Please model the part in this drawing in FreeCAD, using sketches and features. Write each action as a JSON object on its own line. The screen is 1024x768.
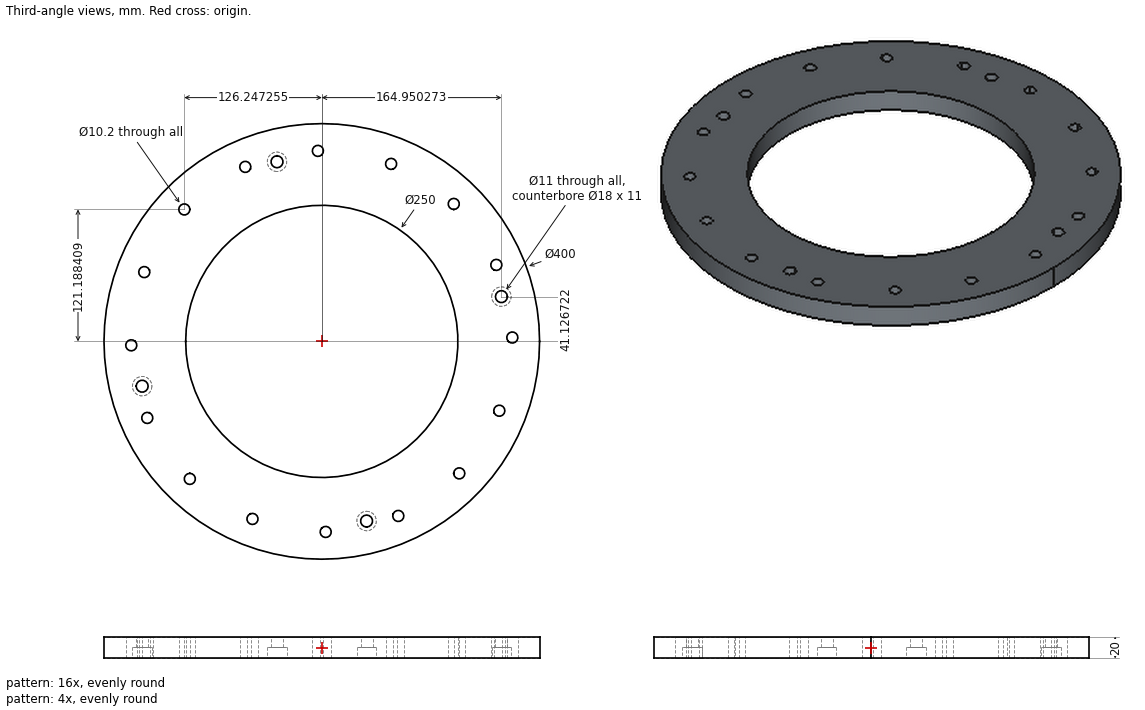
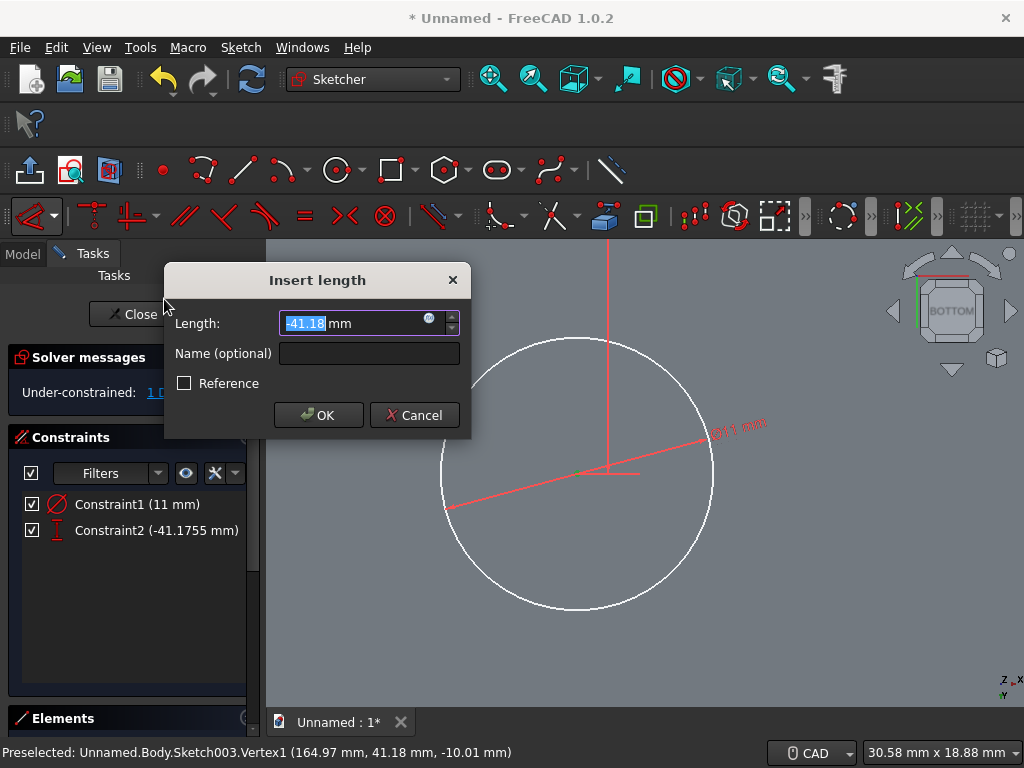
{"action": "type", "text": "-41.126722"}
{"action": "key", "text": "Return"}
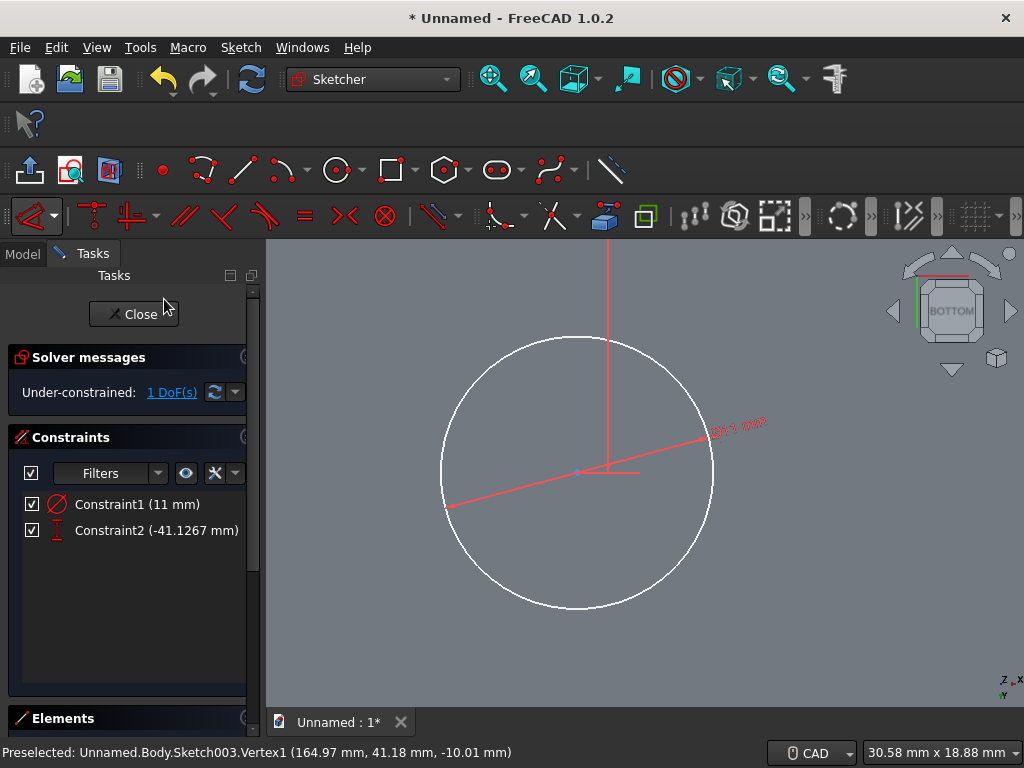
{"action": "left_click", "coordinate": [577, 473]}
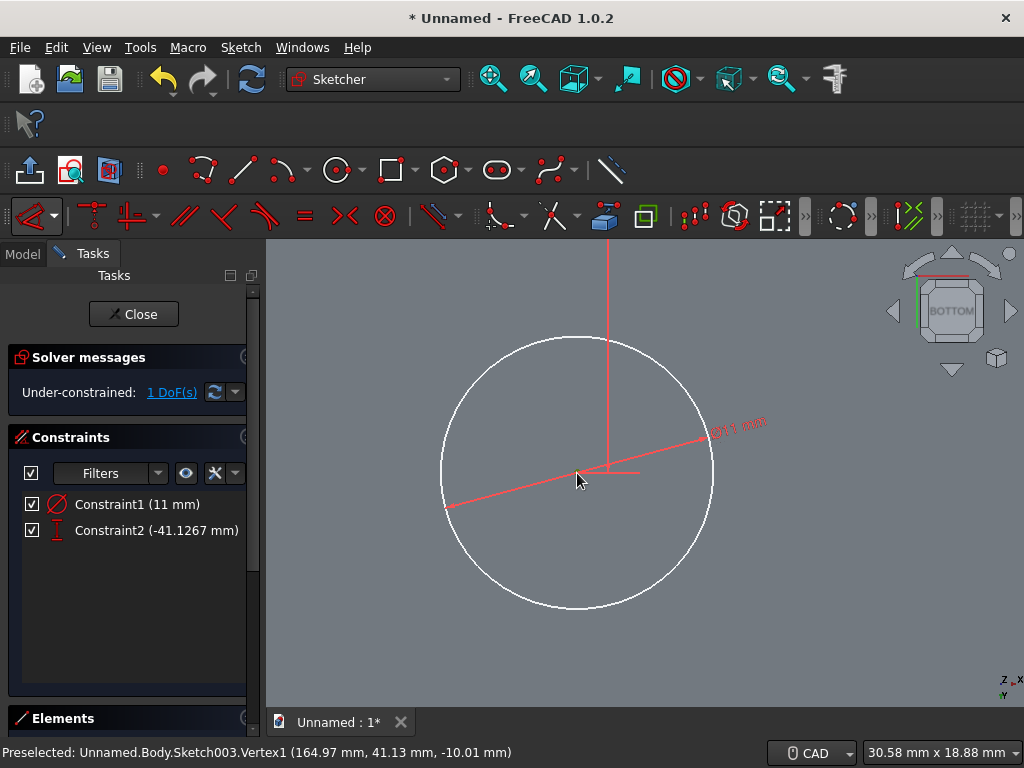
{"action": "key", "text": "l"}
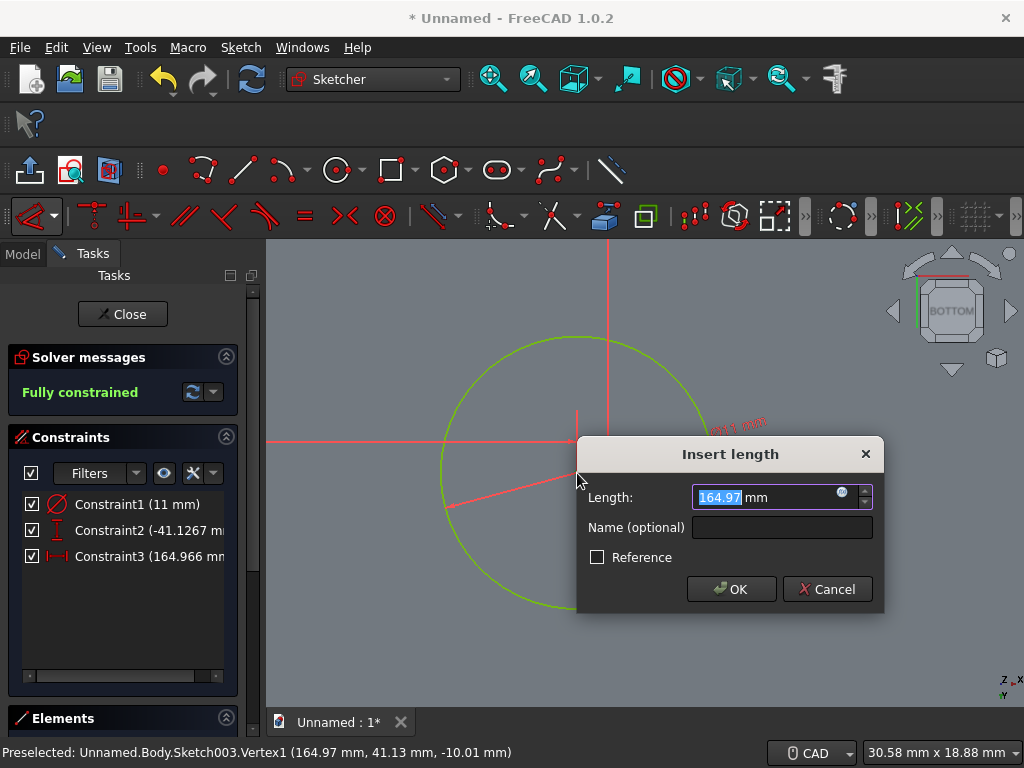
{"action": "type", "text": "164.950273"}
{"action": "key", "text": "Return"}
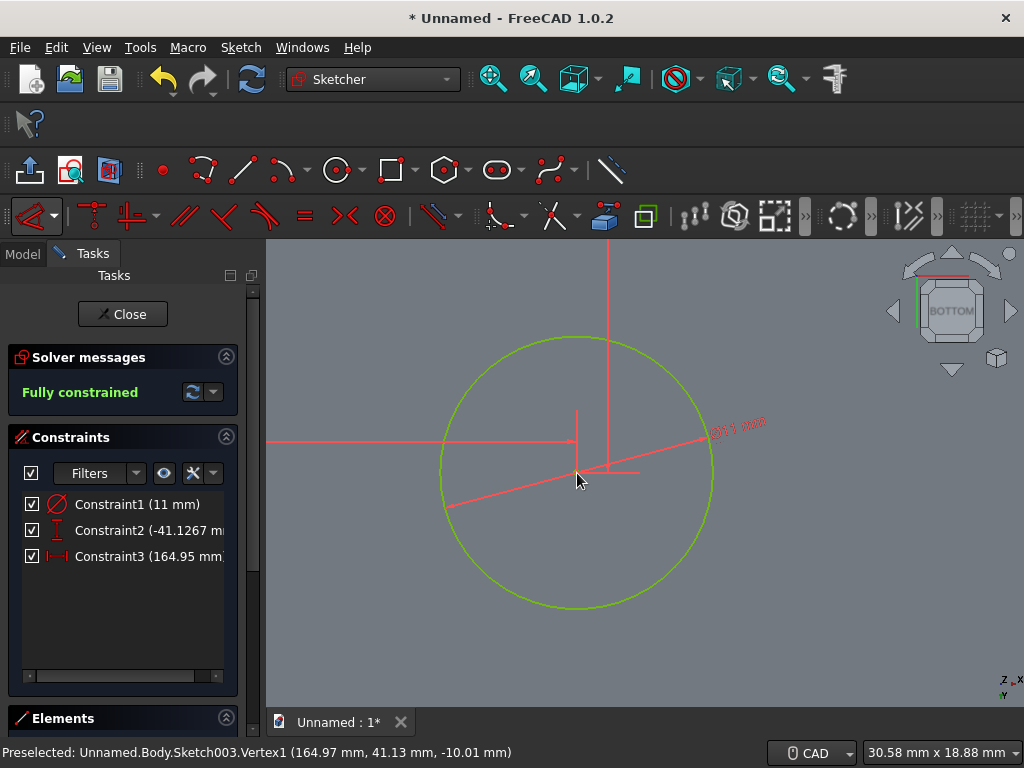
{"action": "left_click", "coordinate": [123, 314]}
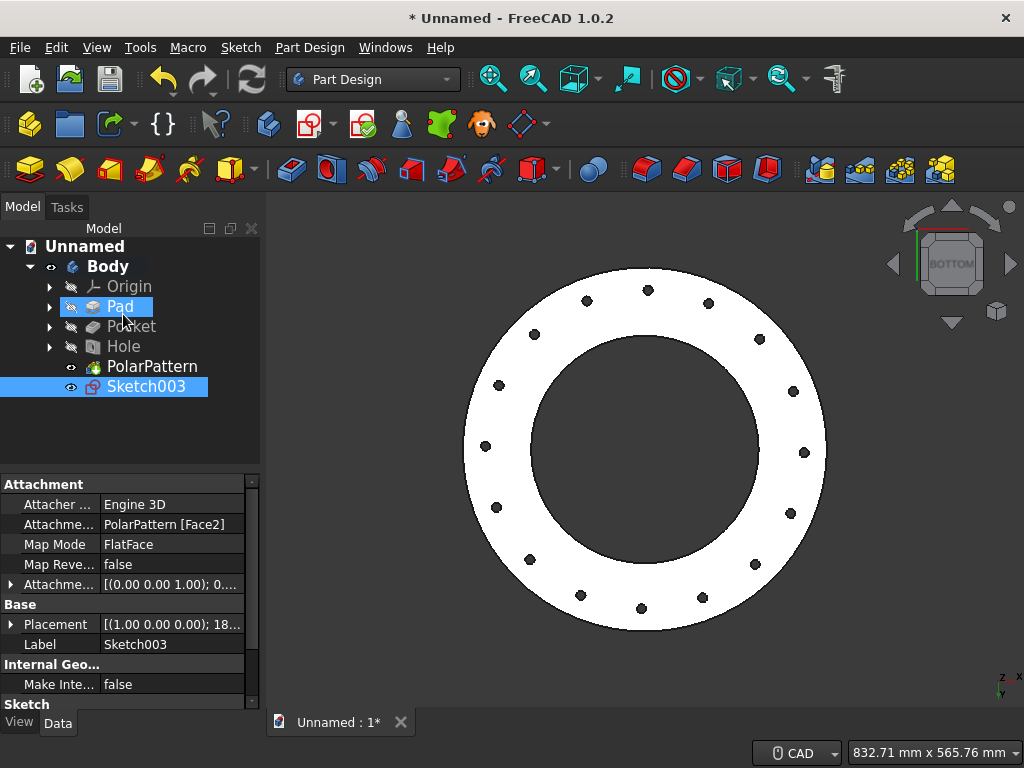
{"action": "left_click", "coordinate": [332, 170]}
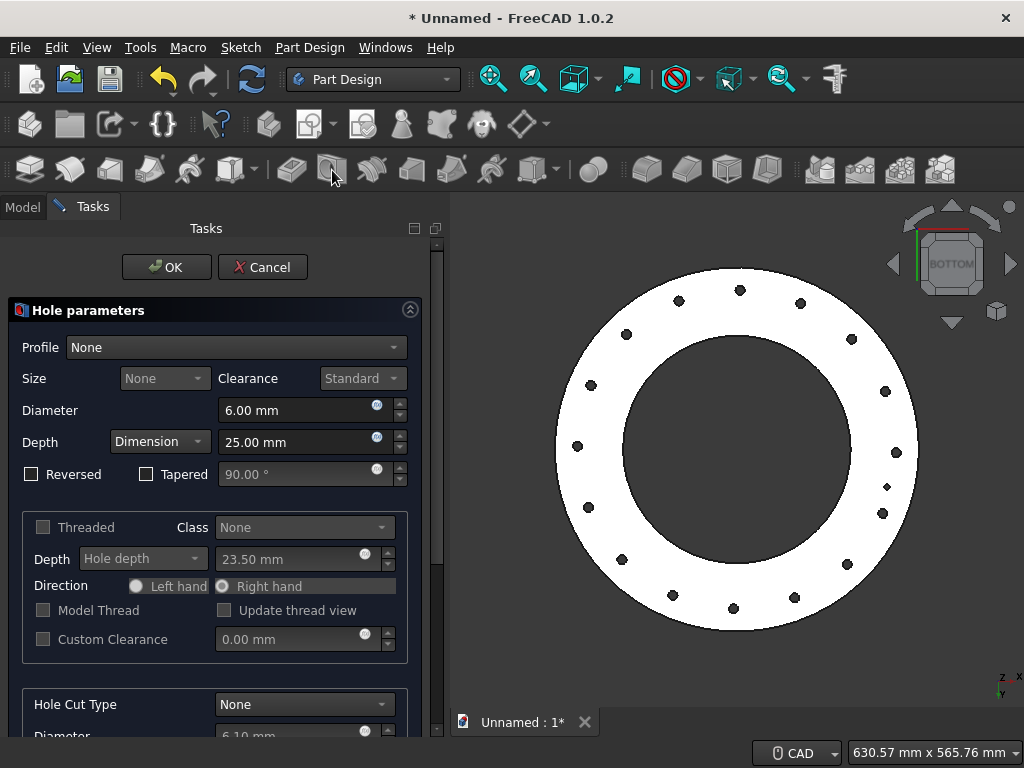
{"action": "triple_click", "coordinate": [305, 410]}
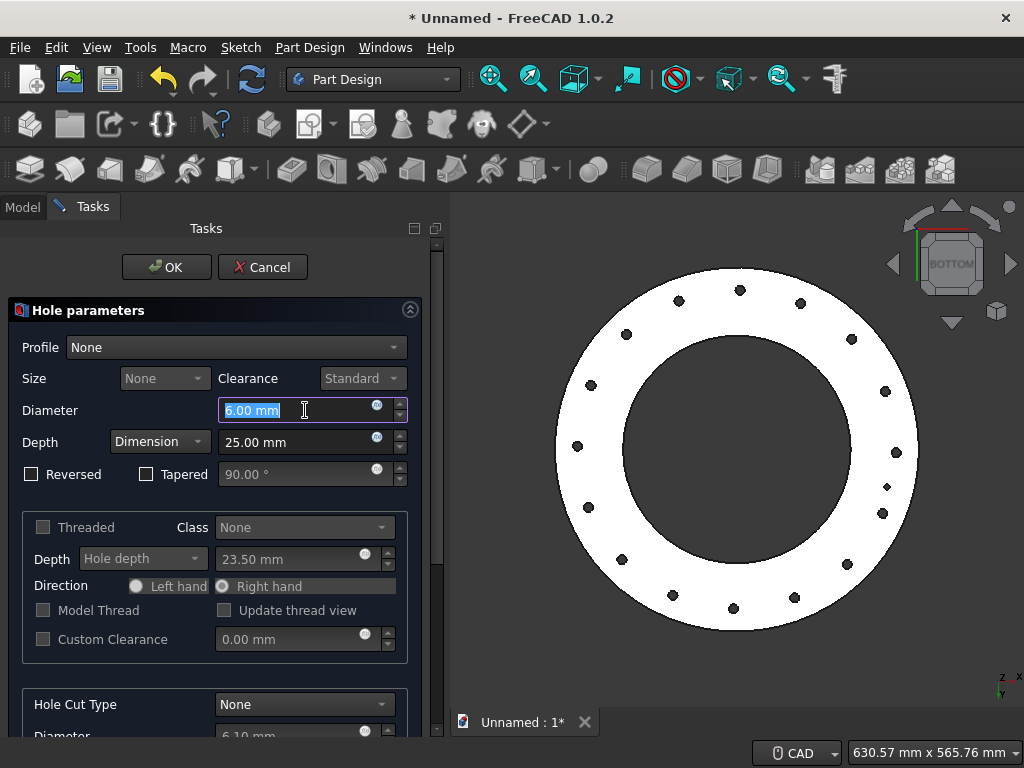
{"action": "type", "text": "11"}
{"action": "key", "text": "Tab"}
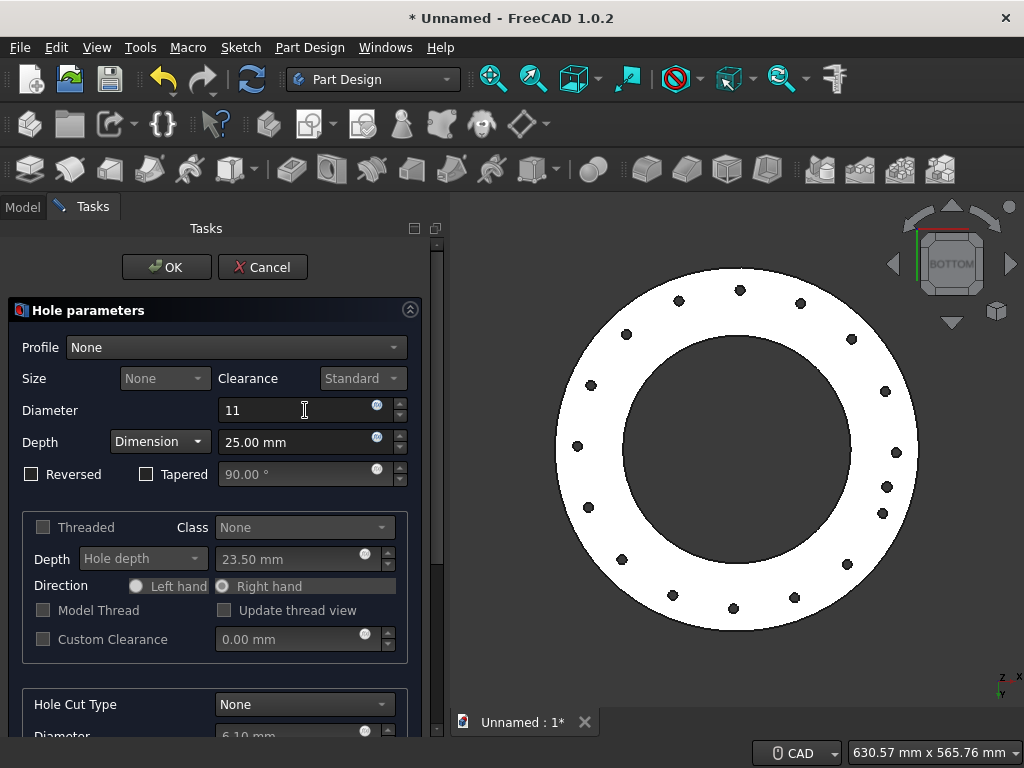
{"action": "left_click", "coordinate": [161, 442]}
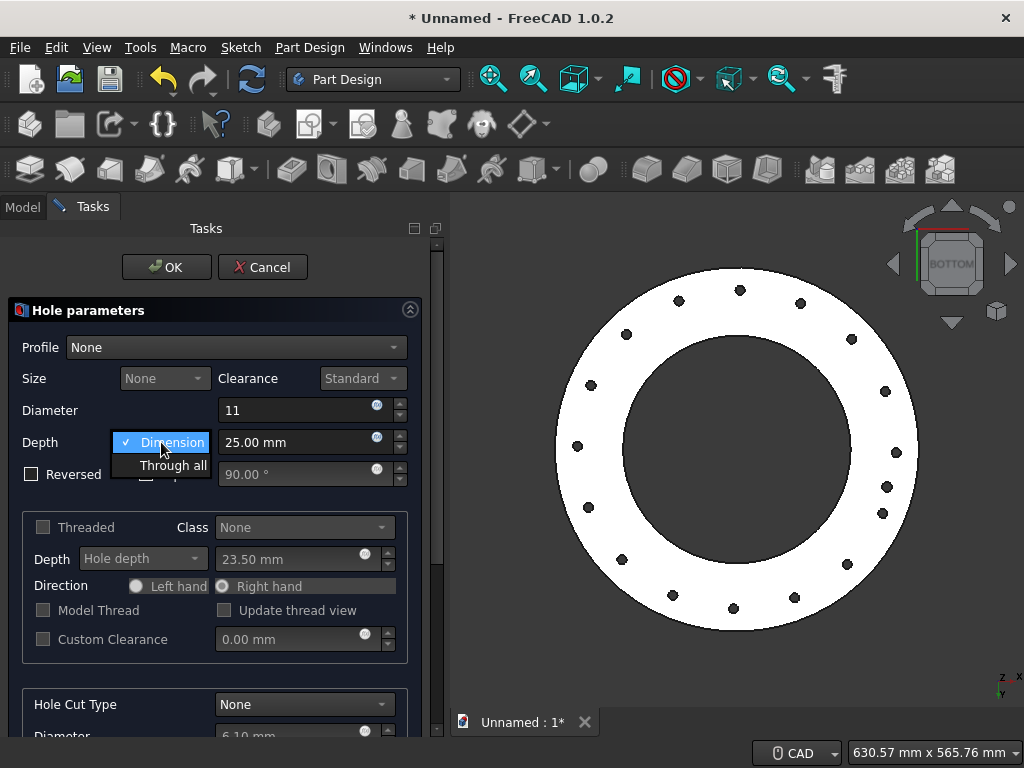
{"action": "left_click", "coordinate": [160, 466]}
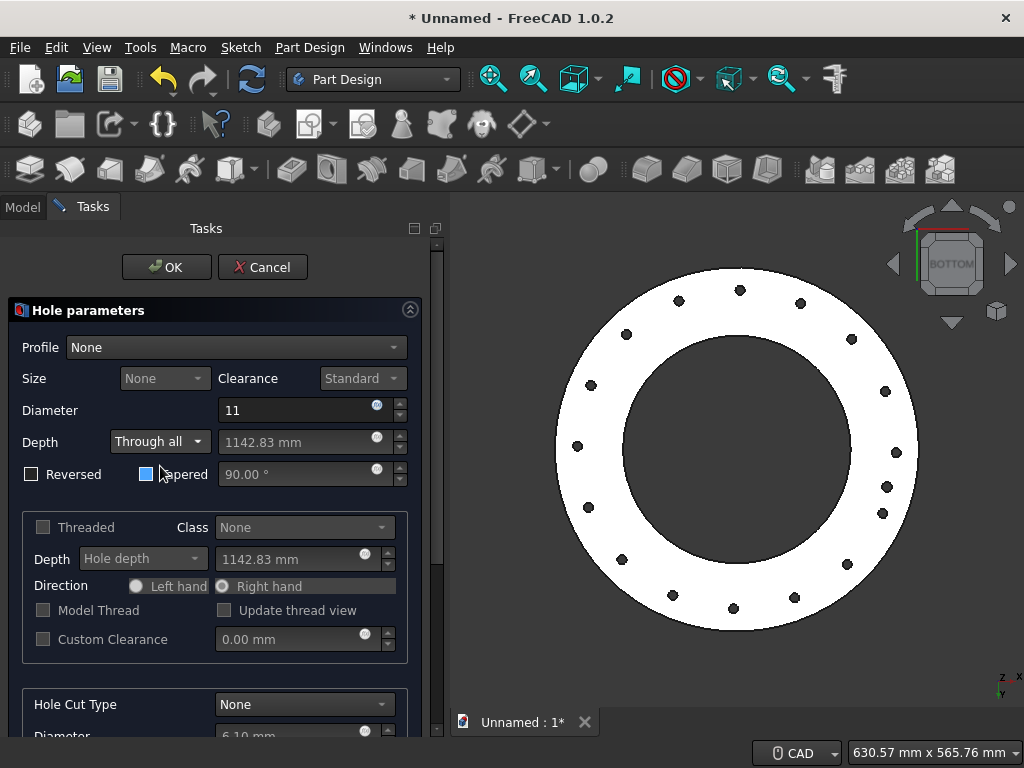
{"action": "left_click", "coordinate": [306, 704]}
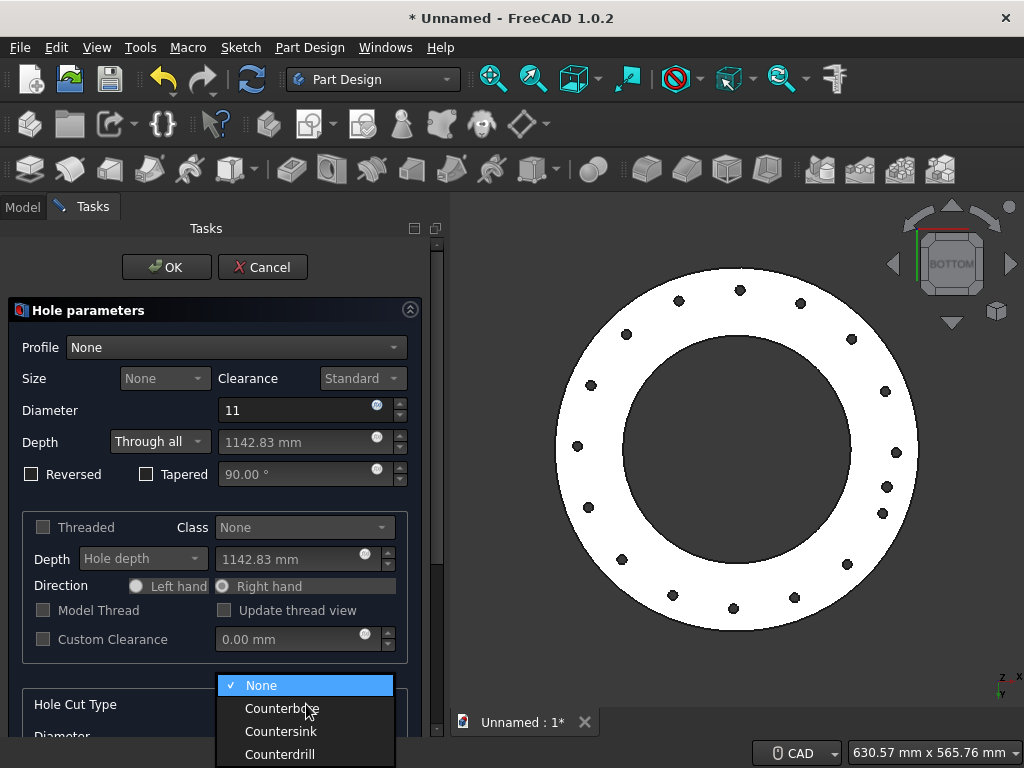
{"action": "left_click", "coordinate": [304, 708]}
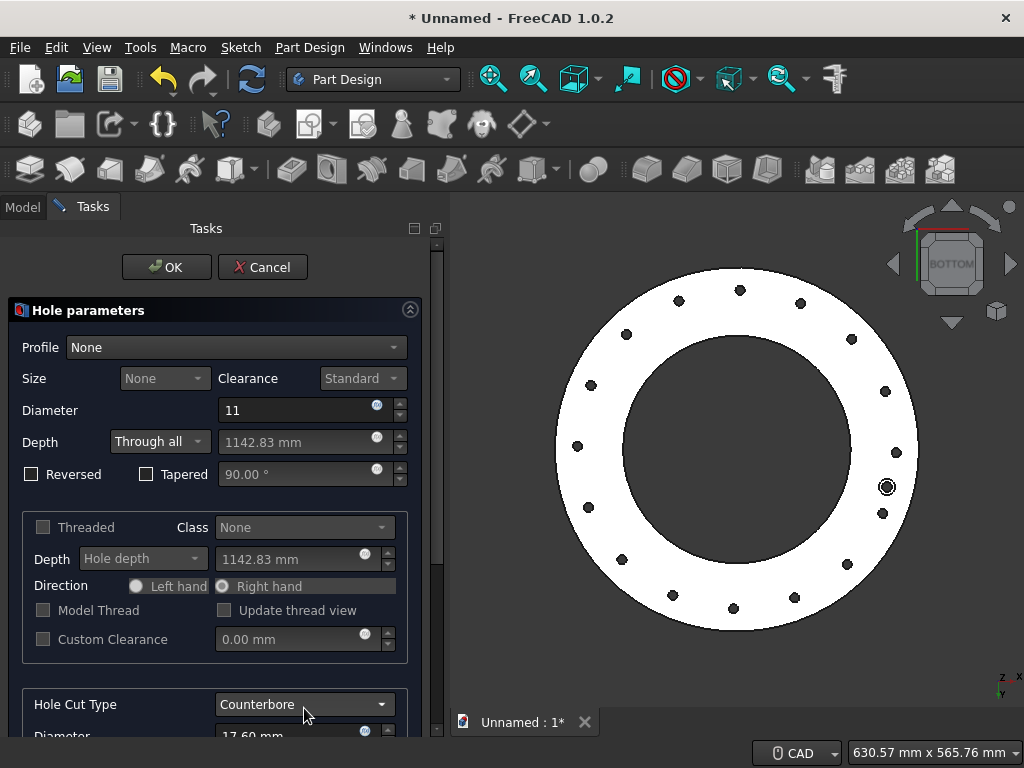
{"action": "scroll", "coordinate": [437, 487], "scroll_direction": "down", "scroll_amount": 2}